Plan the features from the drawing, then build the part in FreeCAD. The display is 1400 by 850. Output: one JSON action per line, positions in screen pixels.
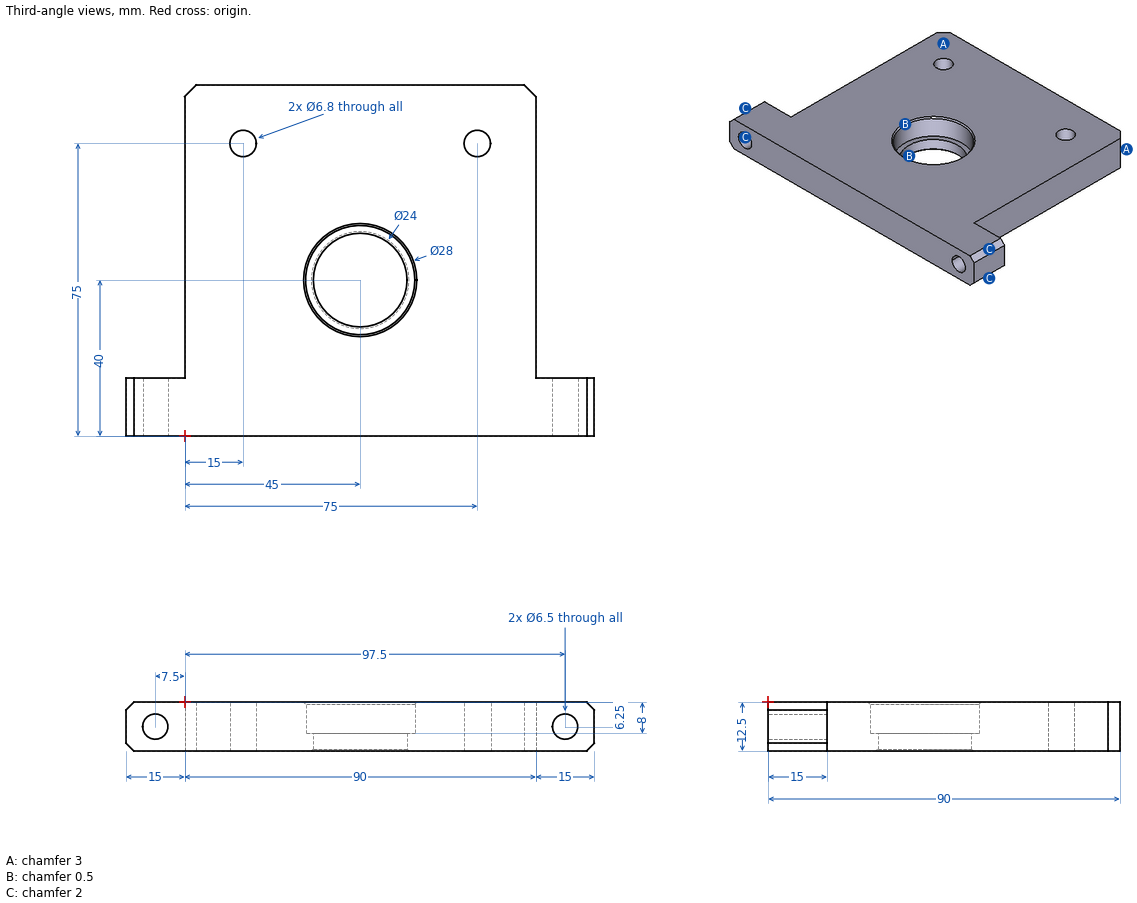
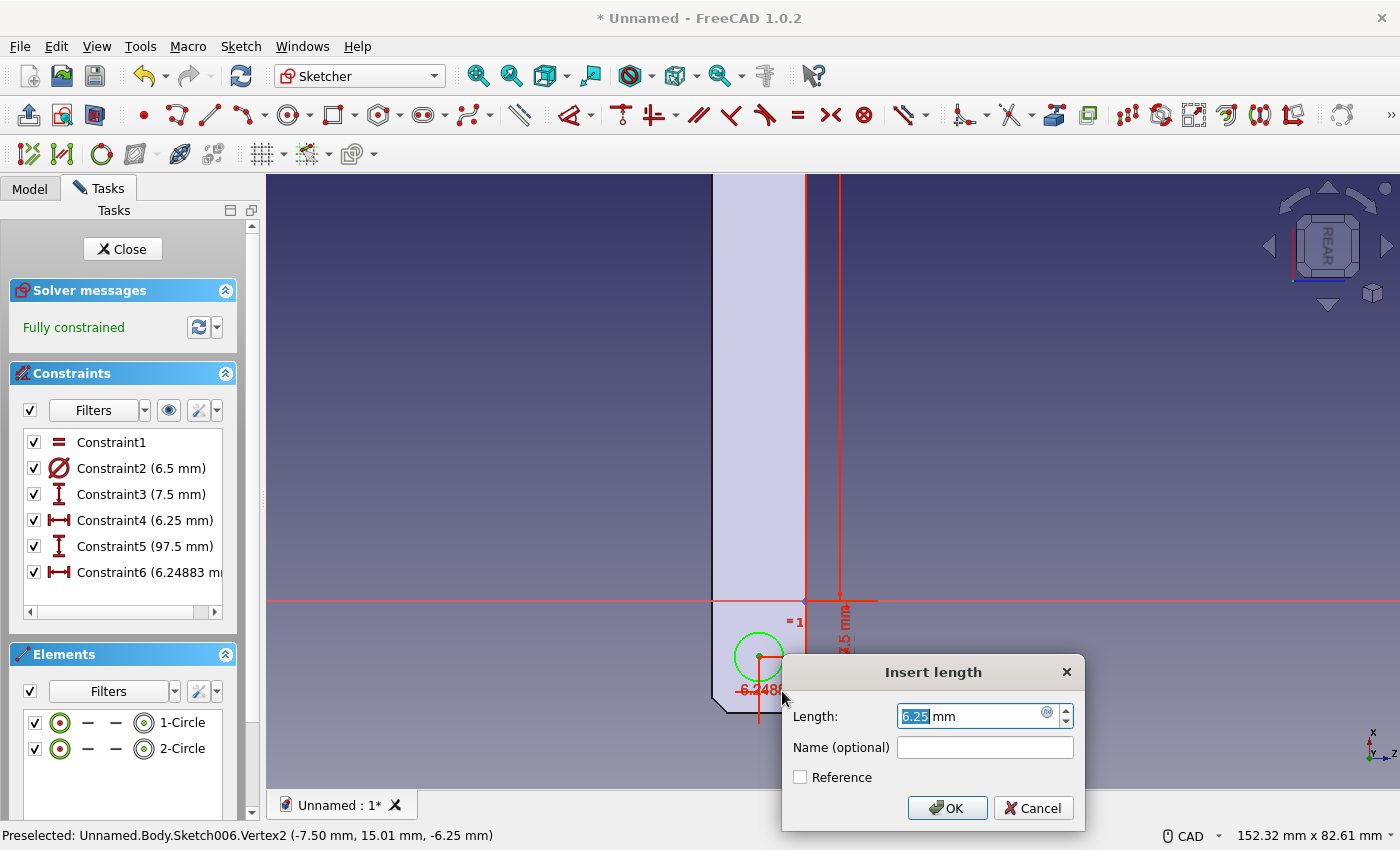
{"action": "type", "text": "6.25"}
{"action": "key", "text": "Return"}
{"action": "key", "text": "Escape"}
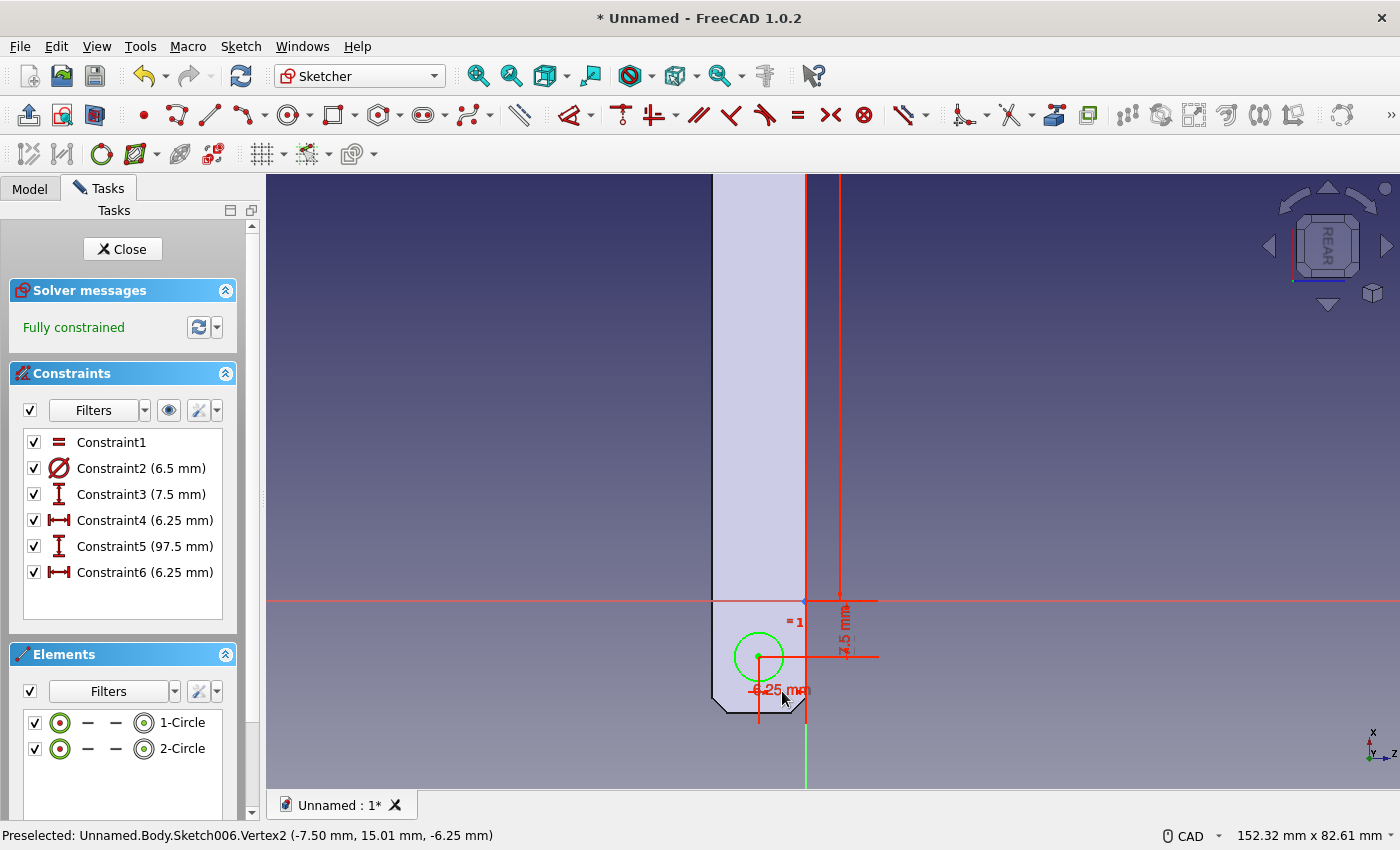
{"action": "left_click", "coordinate": [123, 249]}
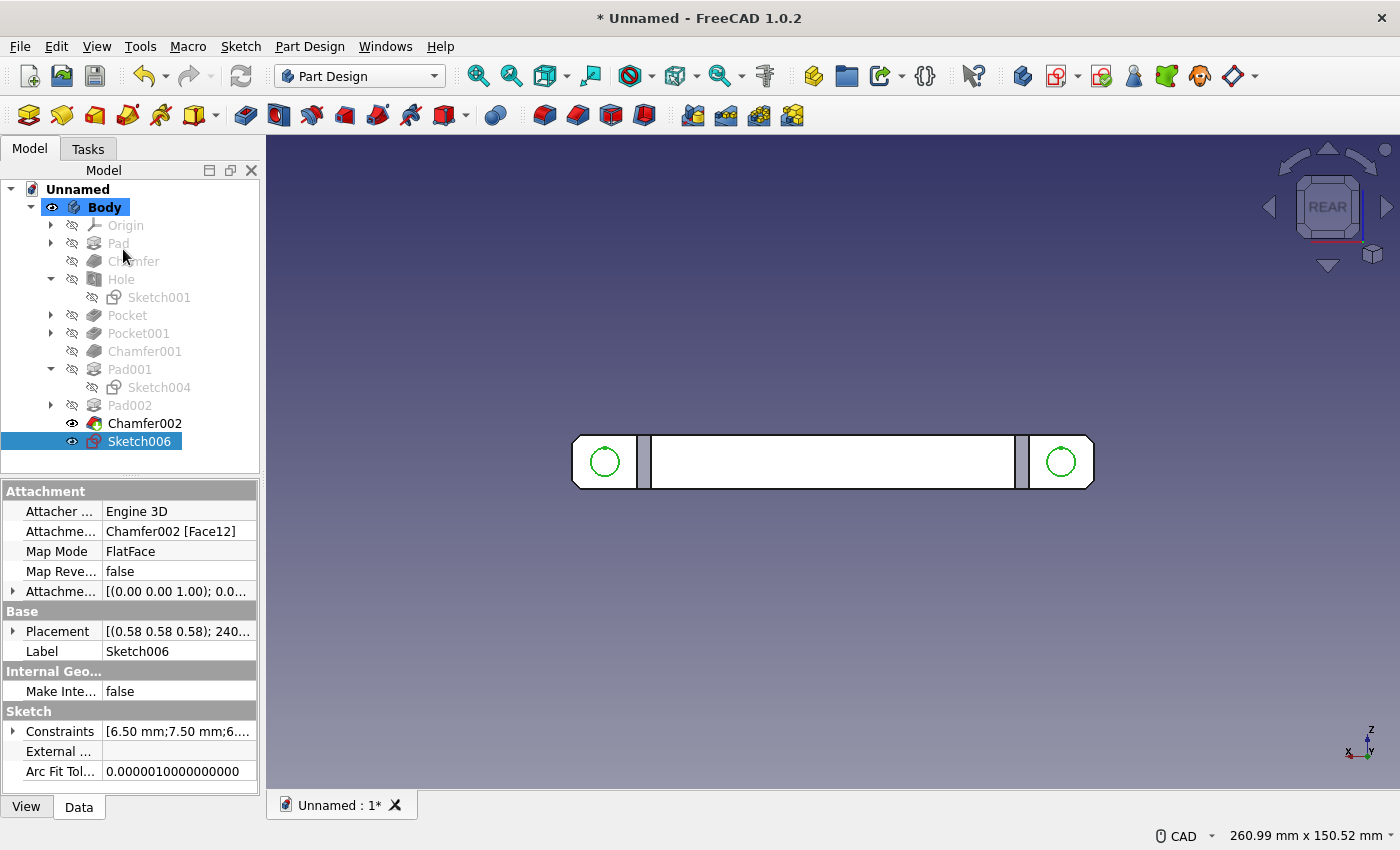
{"action": "left_click", "coordinate": [279, 116]}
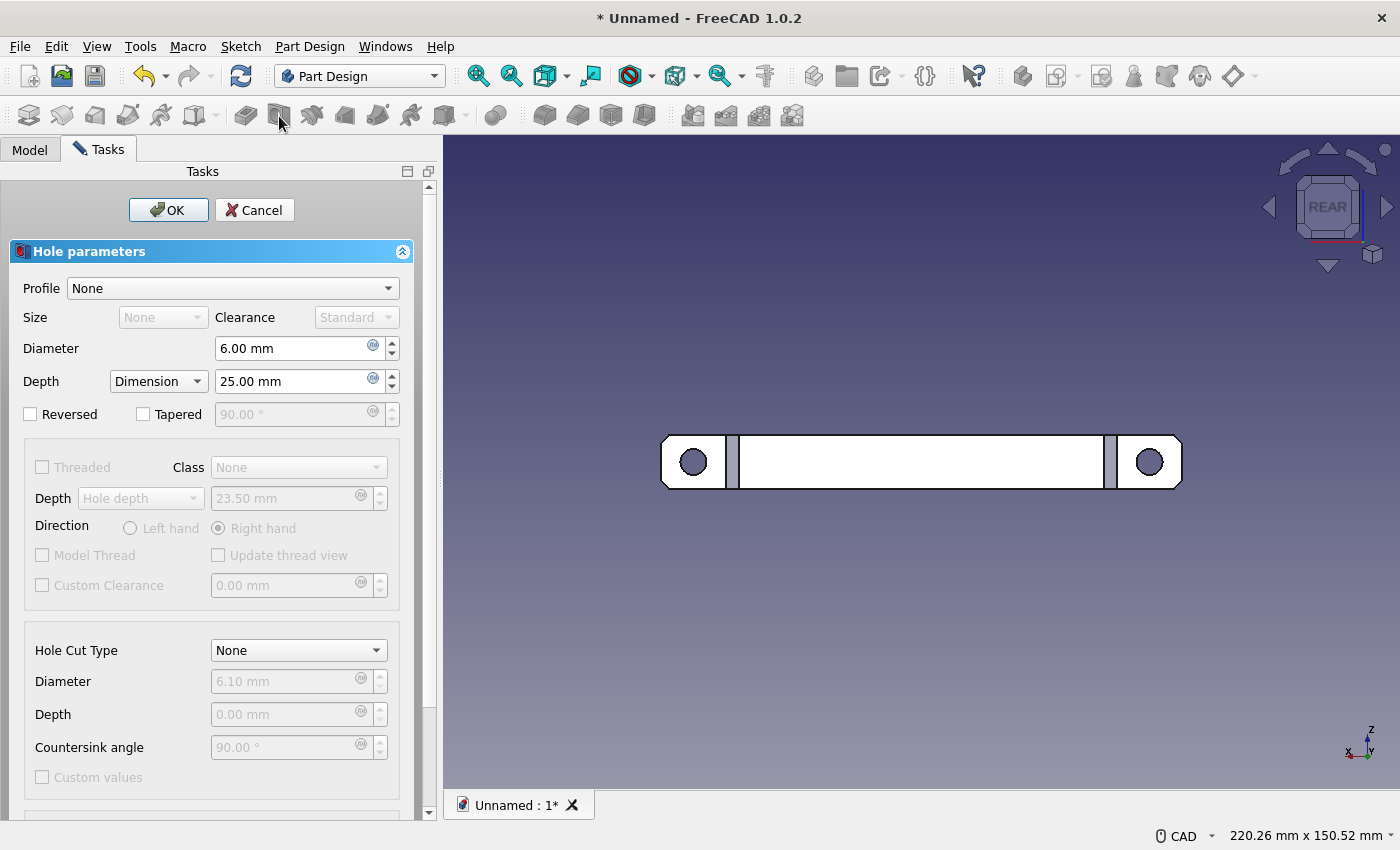
{"action": "triple_click", "coordinate": [300, 348]}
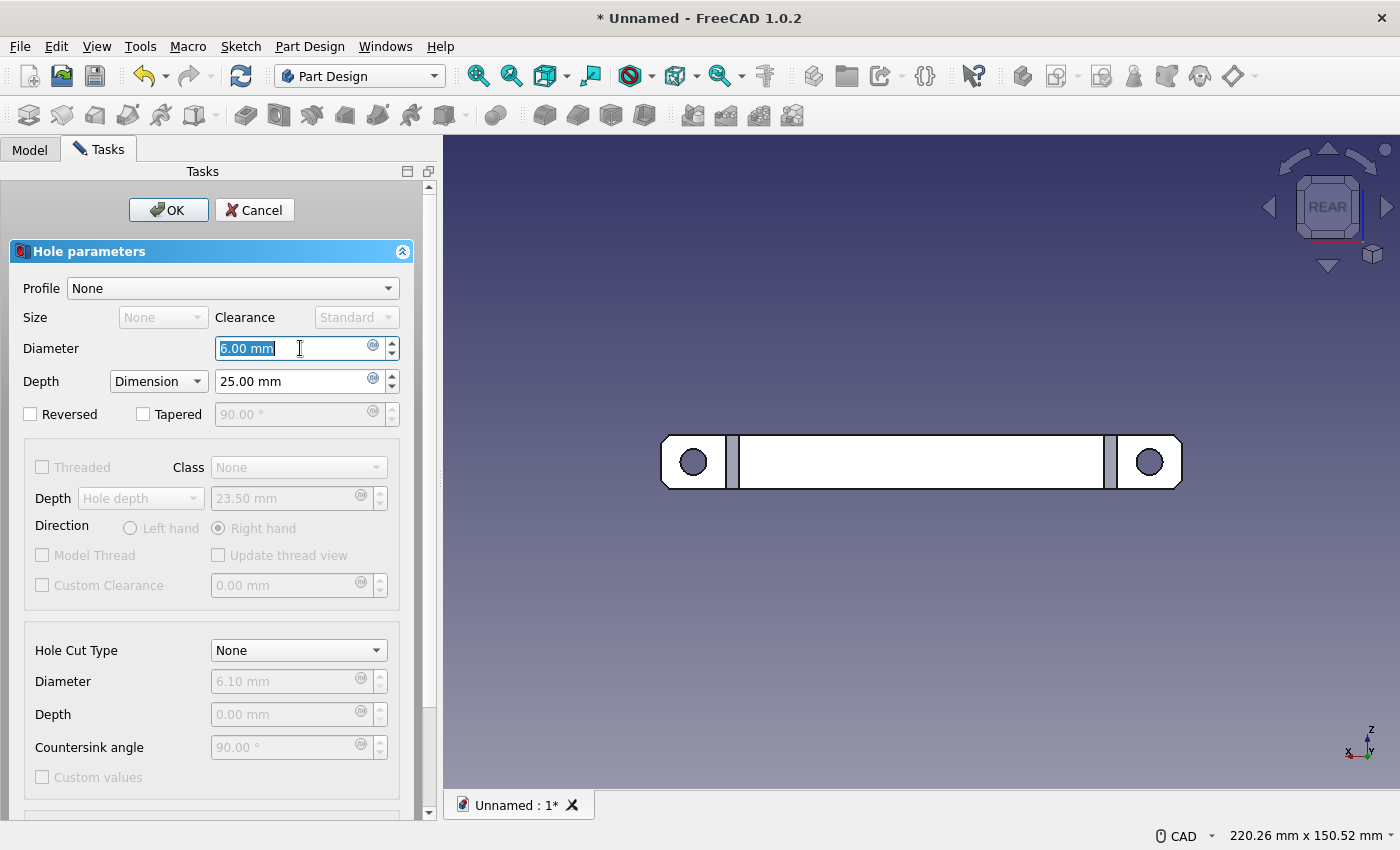
{"action": "type", "text": "6.5"}
{"action": "key", "text": "Tab"}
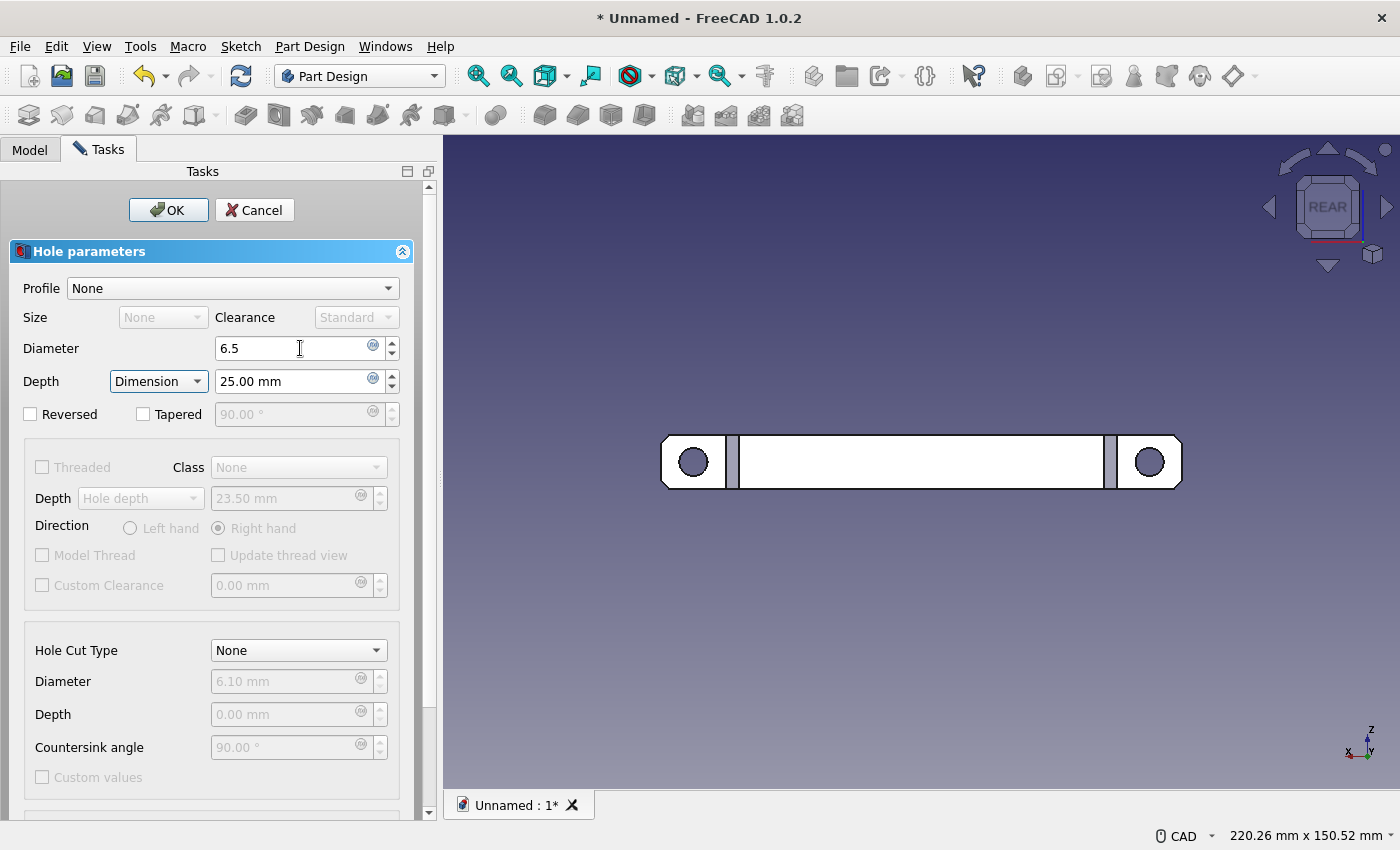
{"action": "left_click", "coordinate": [160, 382]}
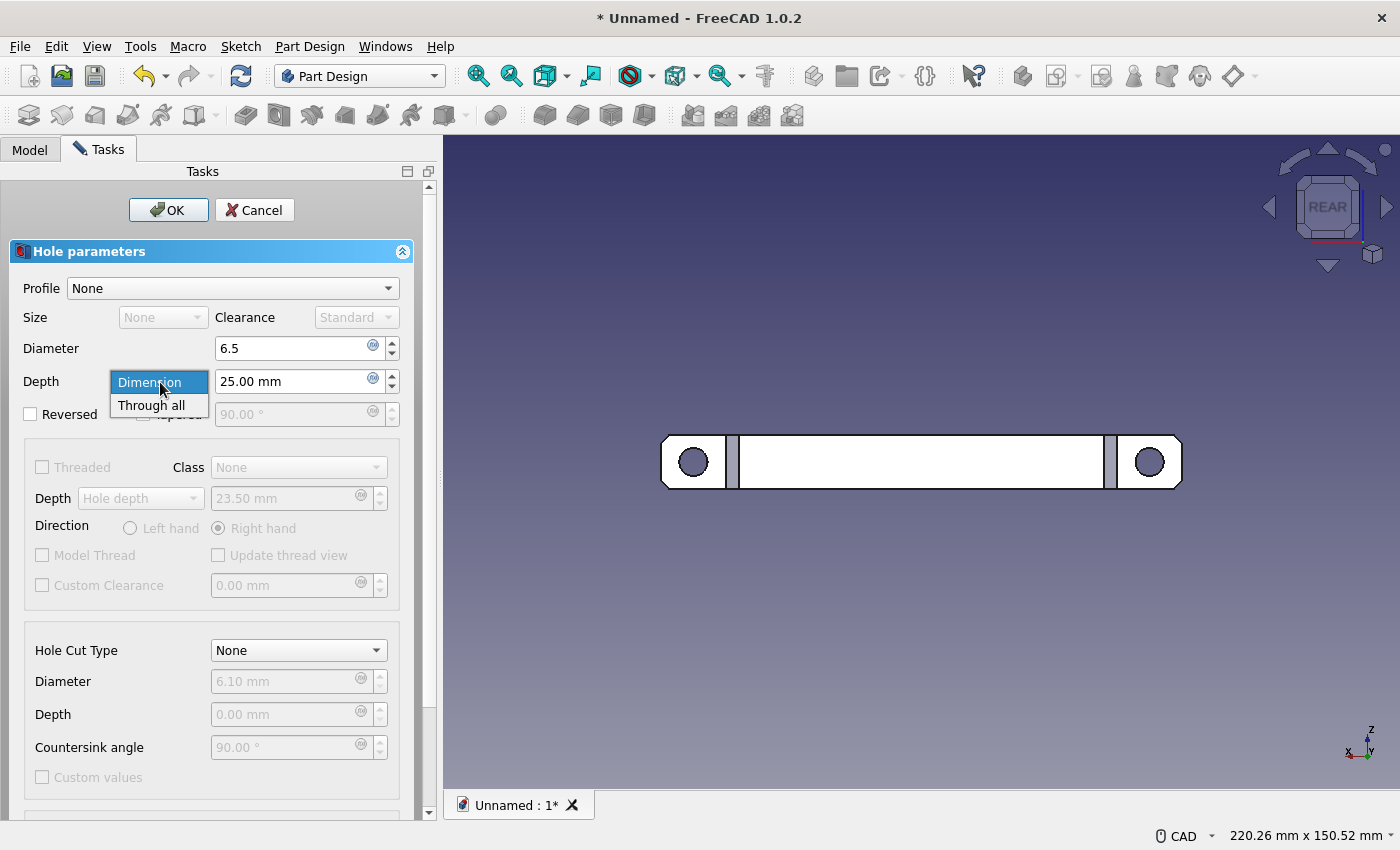
{"action": "left_click", "coordinate": [158, 406]}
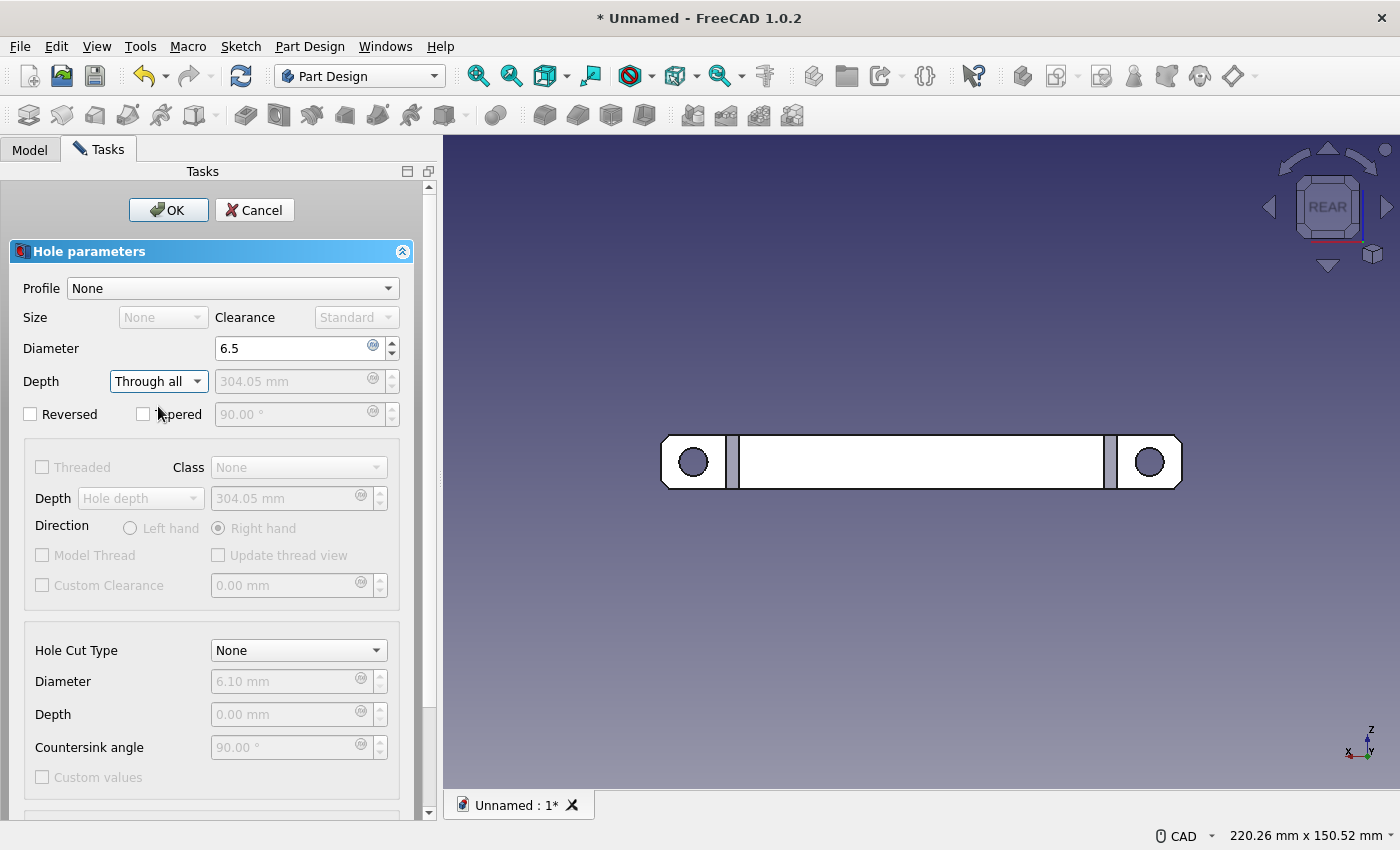
{"action": "left_click", "coordinate": [169, 210]}